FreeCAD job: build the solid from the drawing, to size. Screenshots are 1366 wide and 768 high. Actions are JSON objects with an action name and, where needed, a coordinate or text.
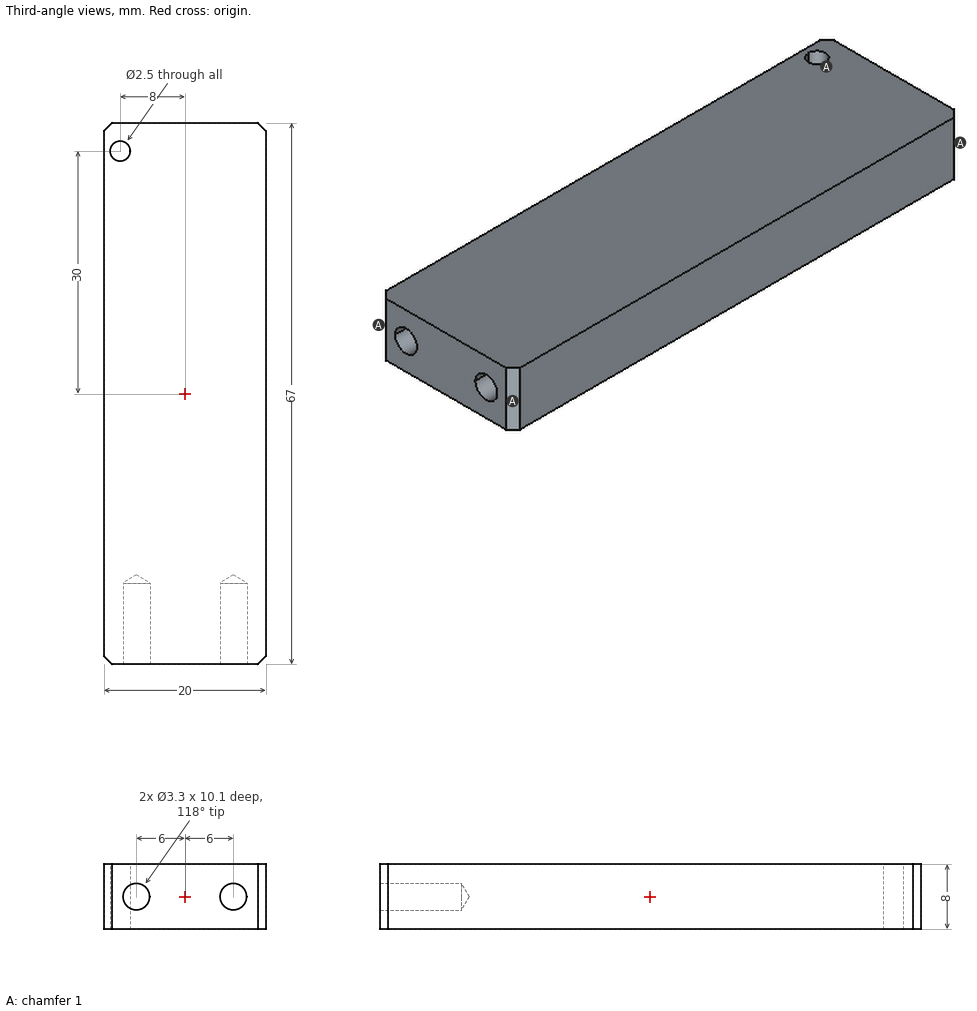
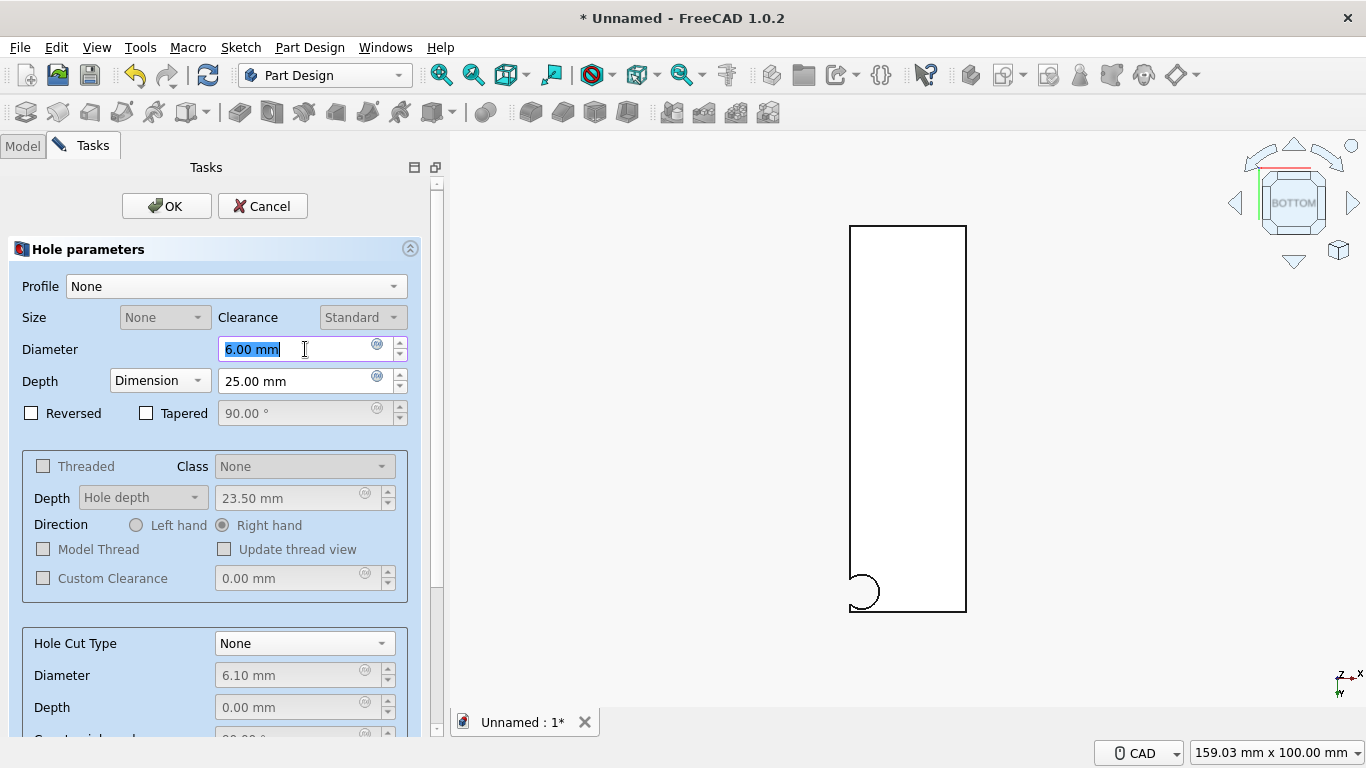
{"action": "type", "text": "2.5"}
{"action": "key", "text": "Tab"}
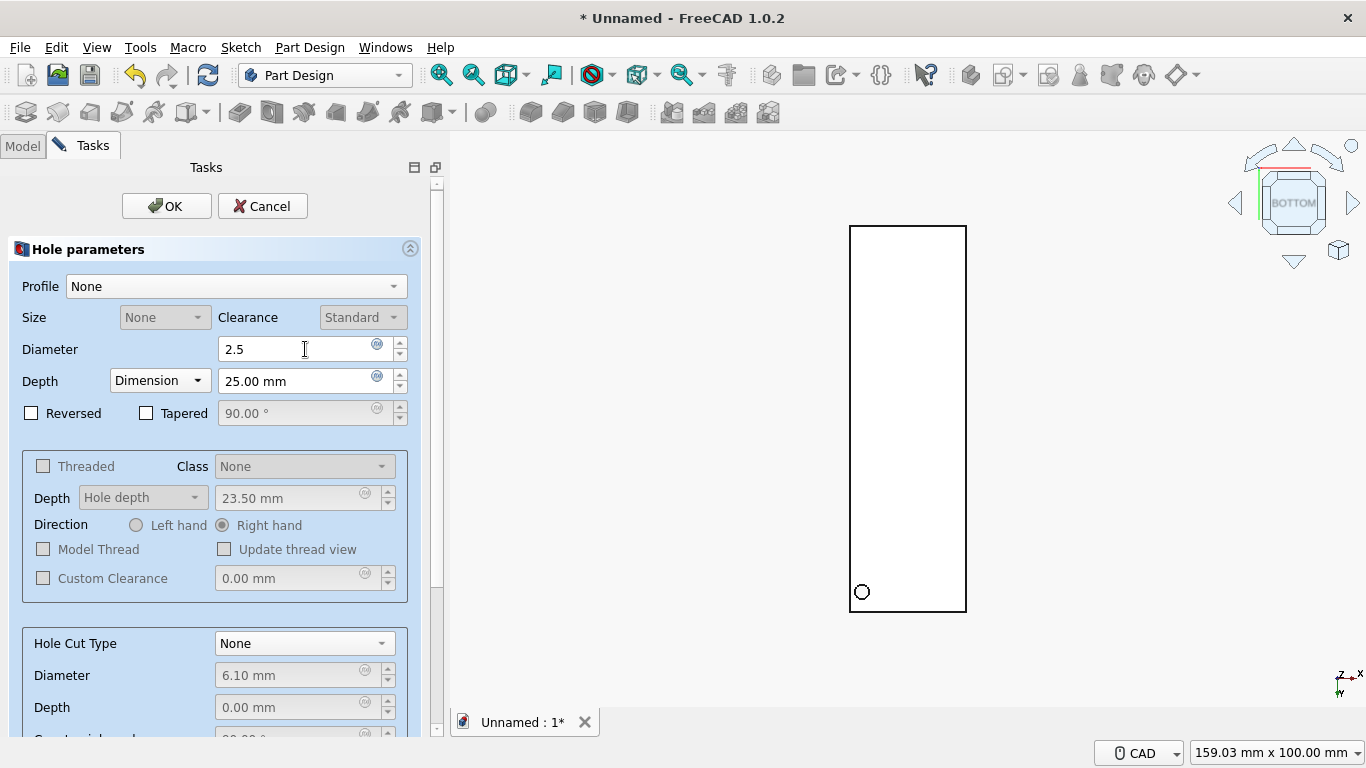
{"action": "left_click", "coordinate": [161, 380]}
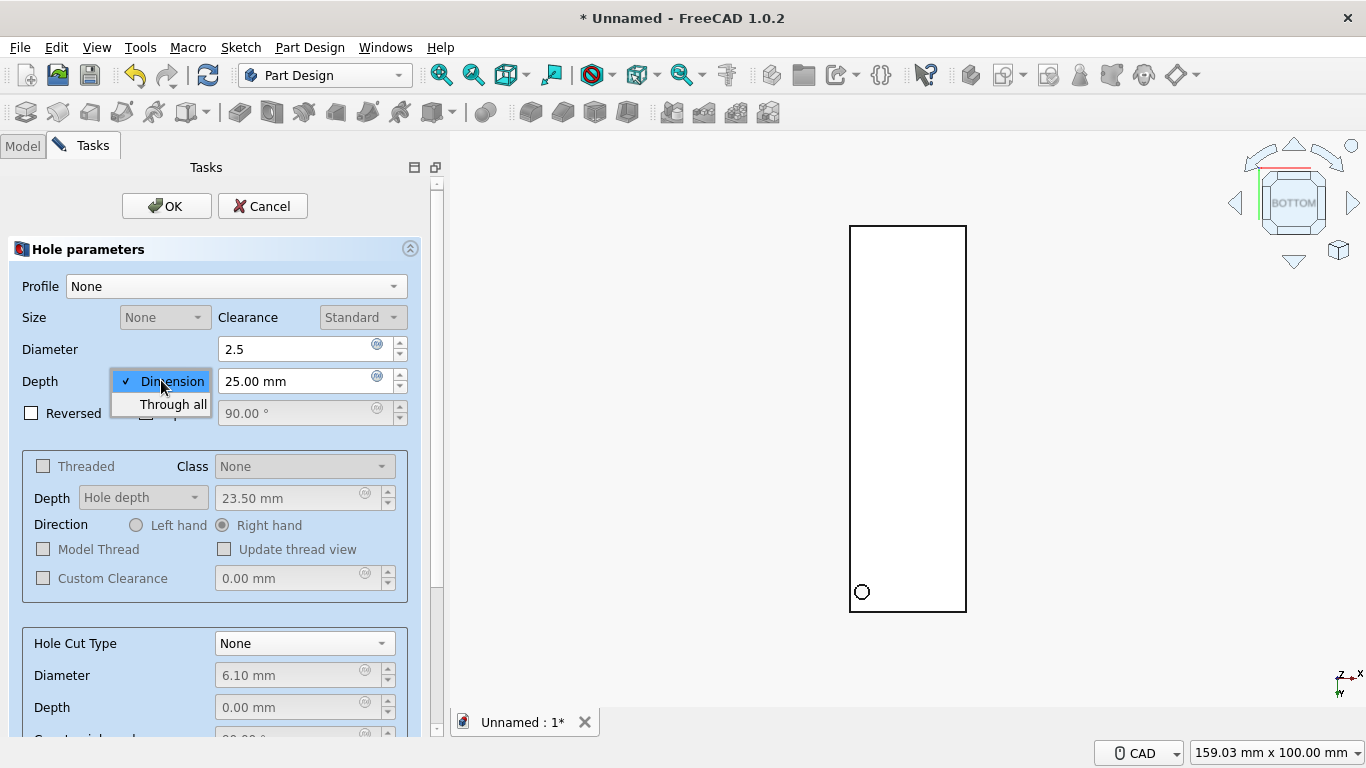
{"action": "left_click", "coordinate": [160, 404]}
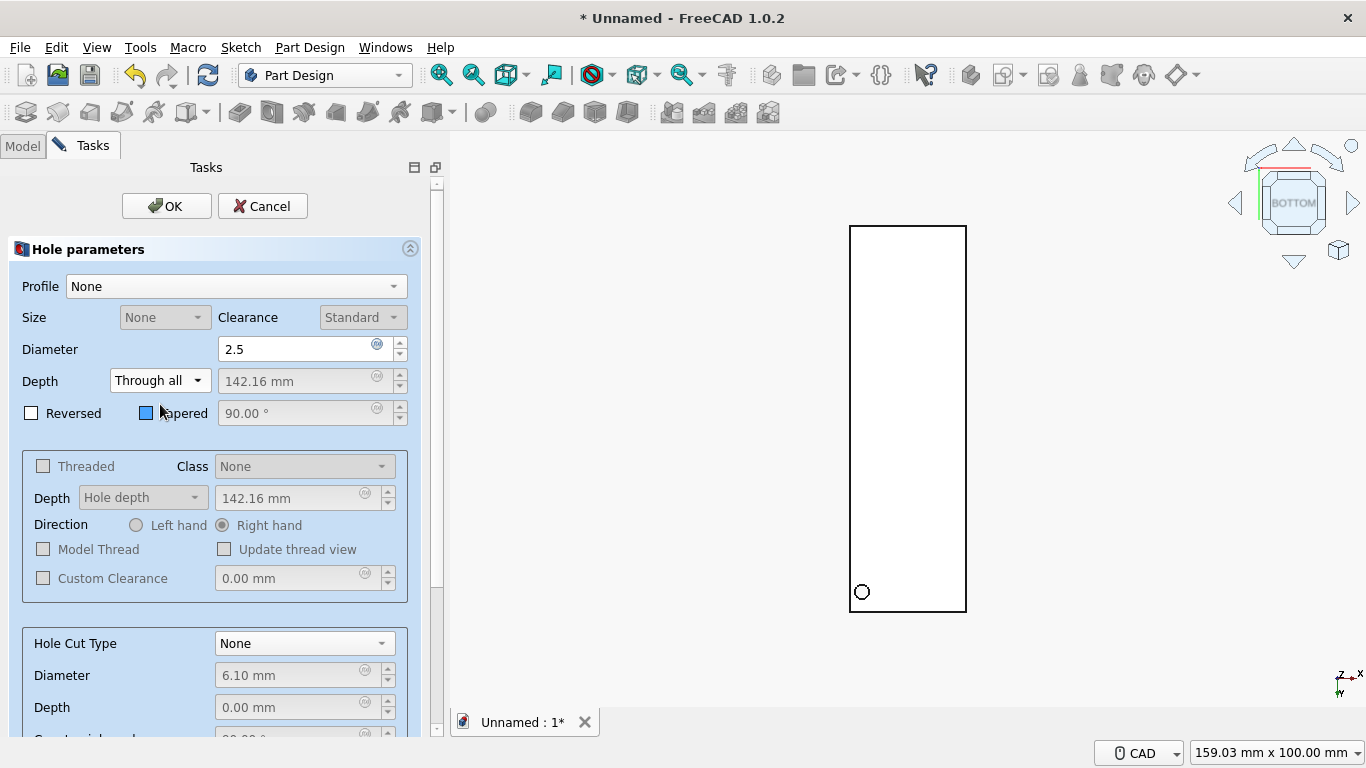
{"action": "left_click", "coordinate": [167, 206]}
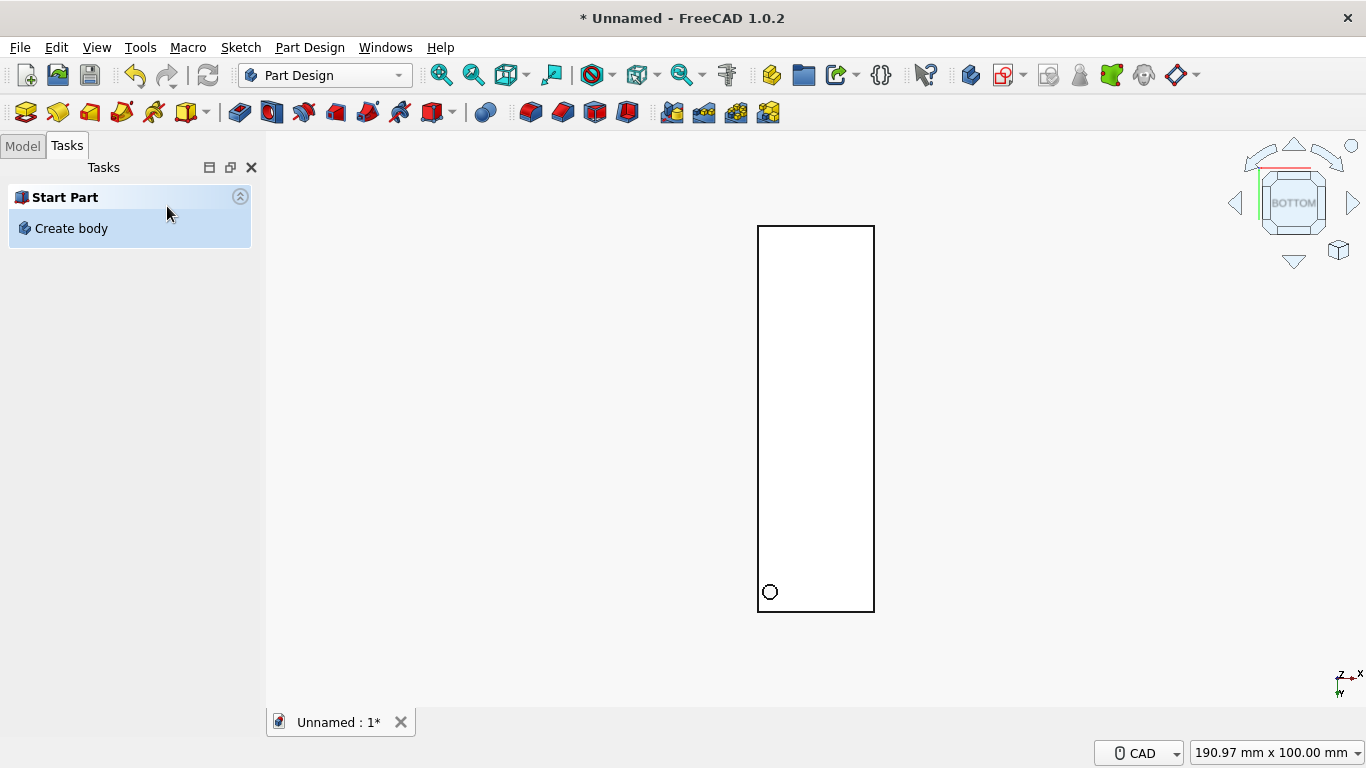
{"action": "key", "text": "0"}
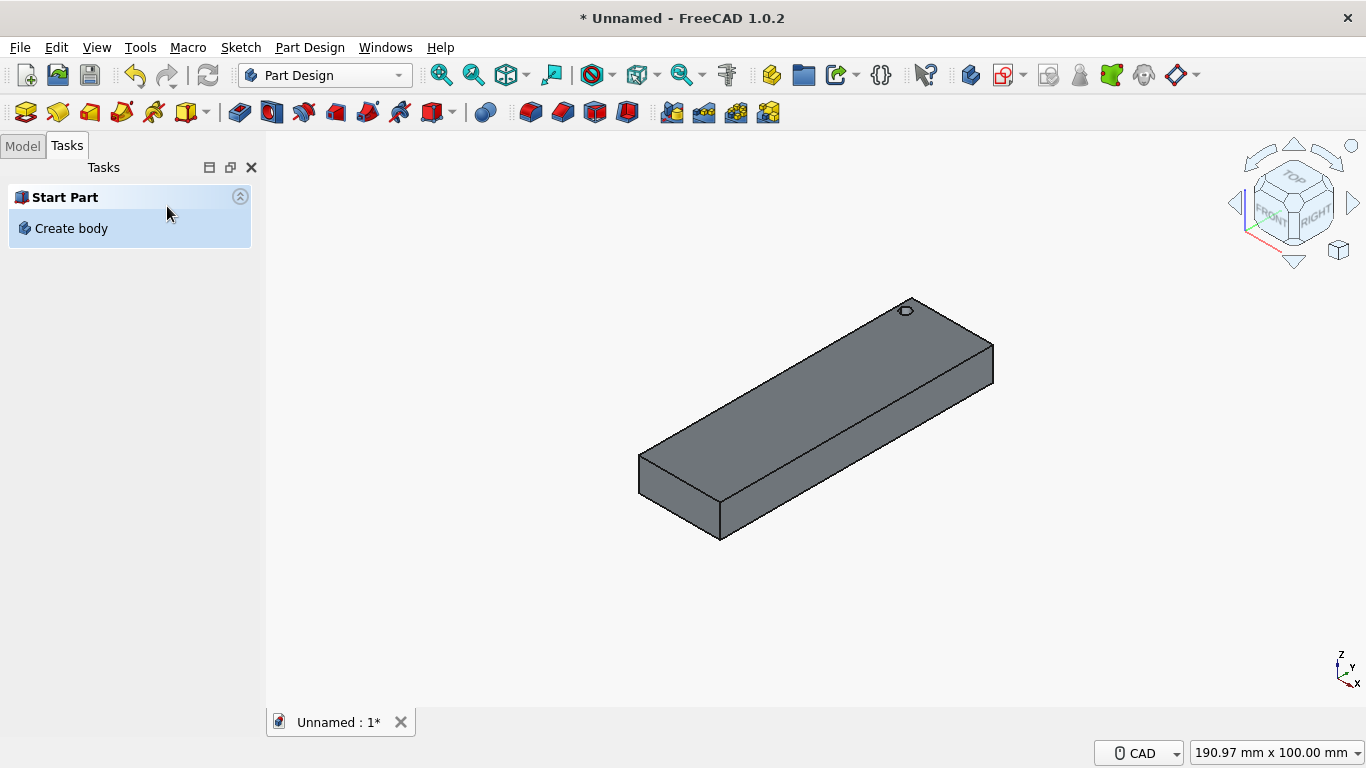
{"action": "key", "text": "v f"}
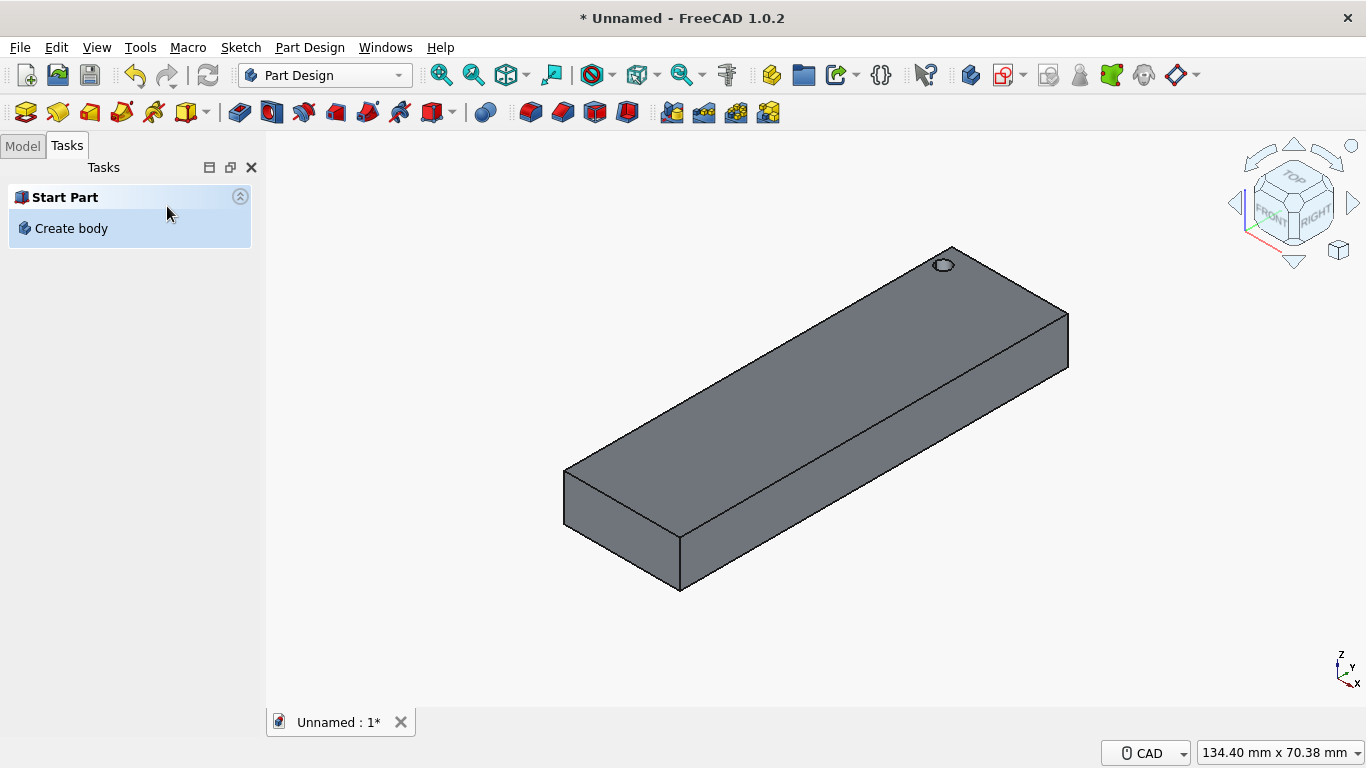
{"action": "left_click", "coordinate": [655, 549]}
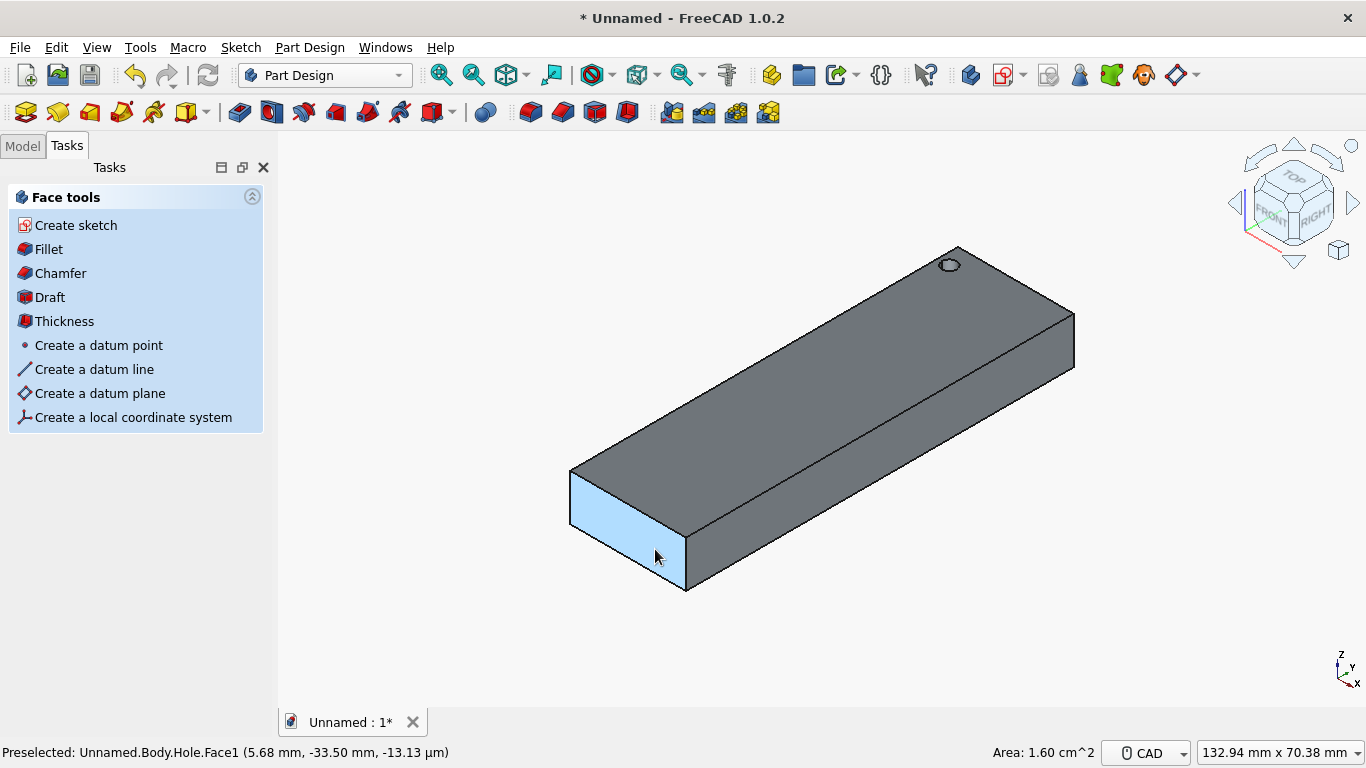
{"action": "left_click", "coordinate": [1004, 76]}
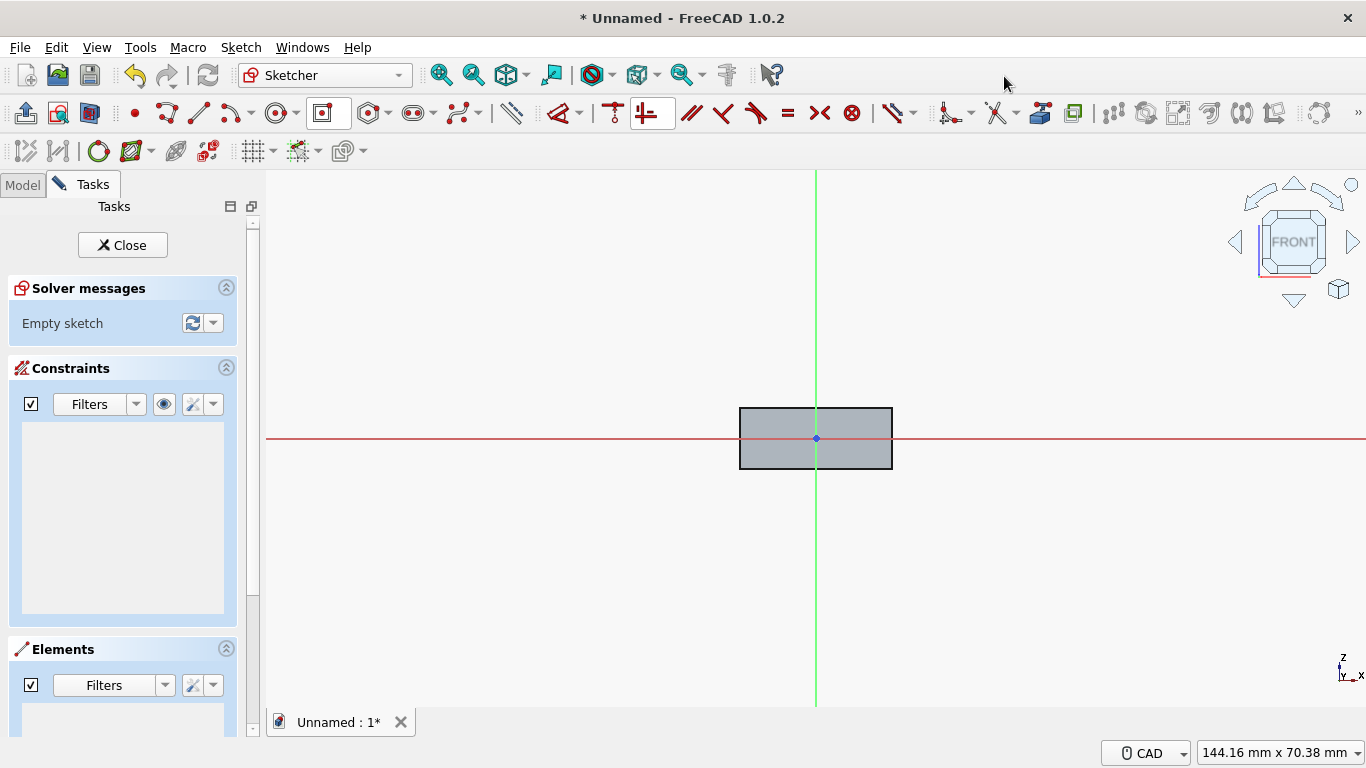
{"action": "scroll", "coordinate": [830, 438], "scroll_direction": "up", "scroll_amount": 9}